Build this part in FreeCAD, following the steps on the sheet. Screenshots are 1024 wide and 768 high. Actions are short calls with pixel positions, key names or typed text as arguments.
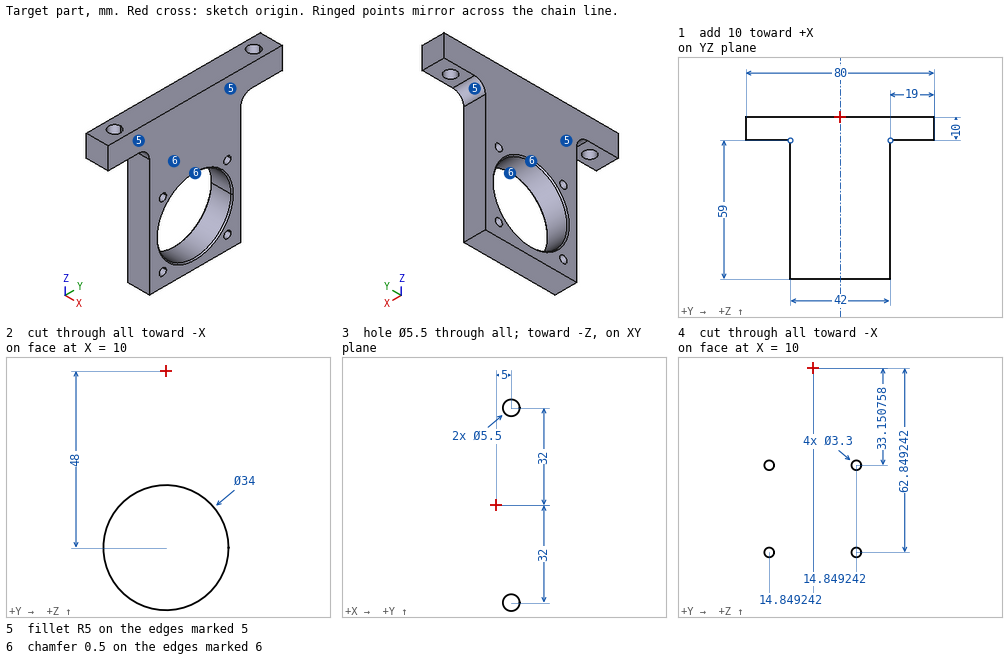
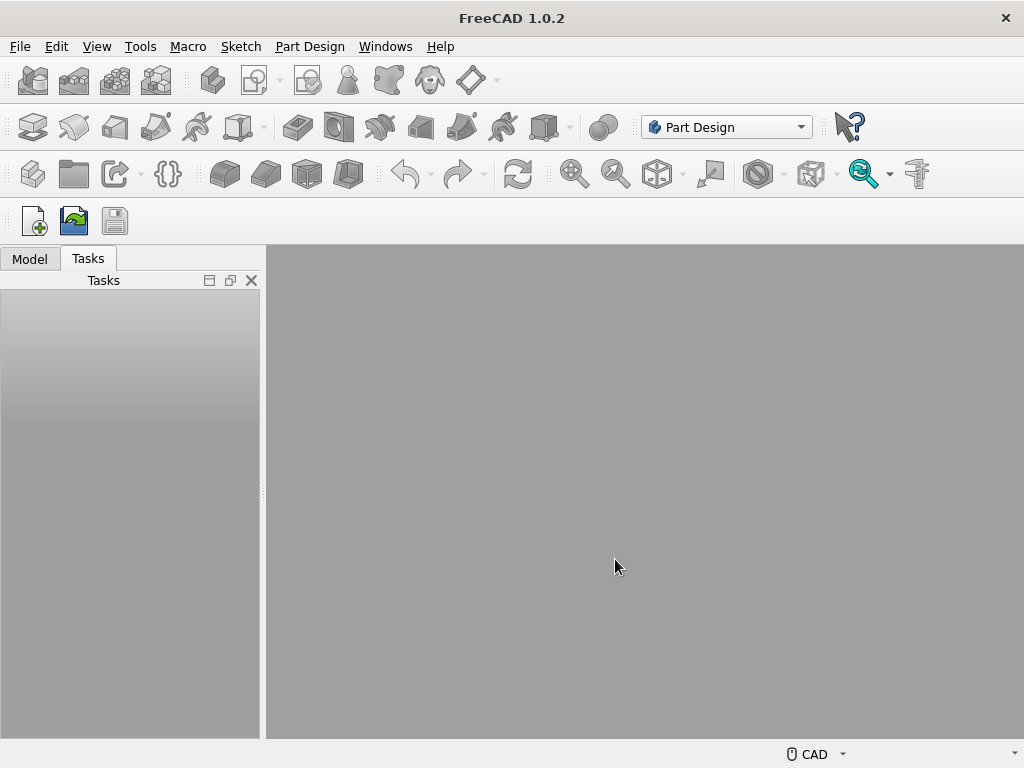
click(33, 222)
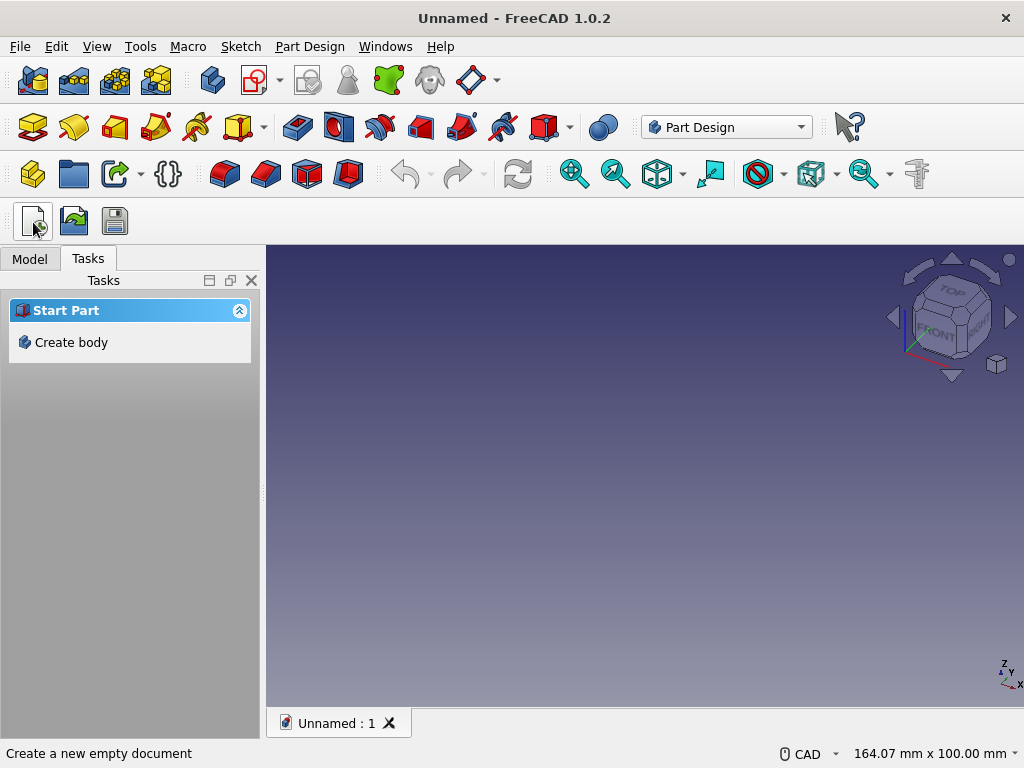
click(254, 80)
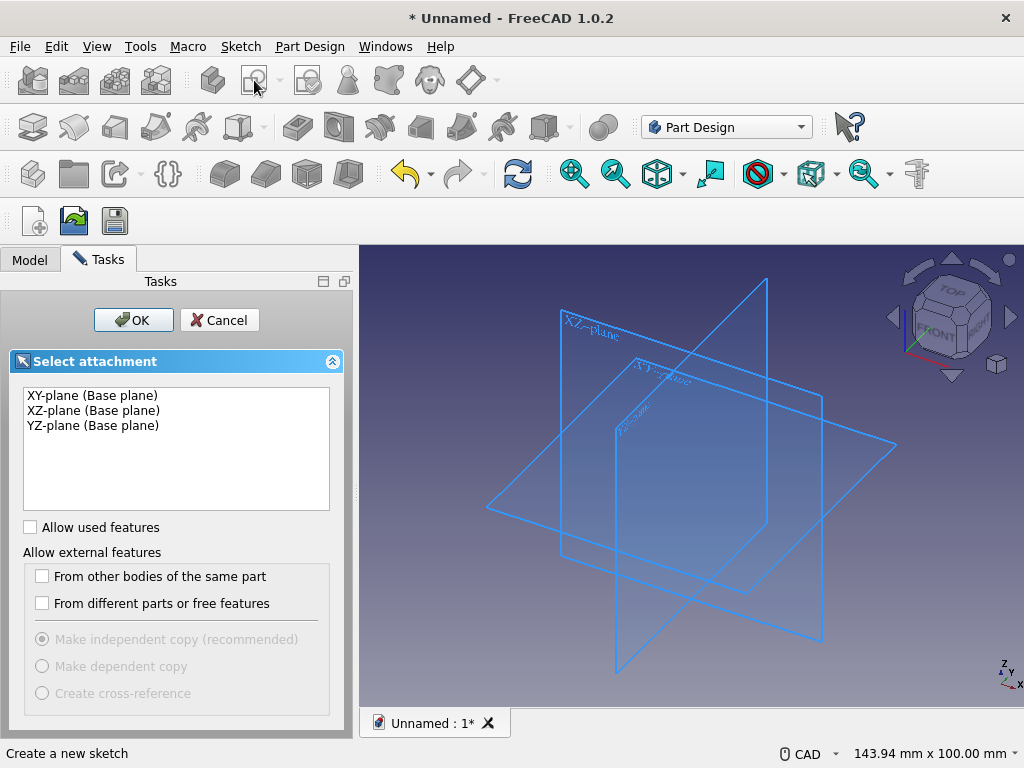
click(84, 426)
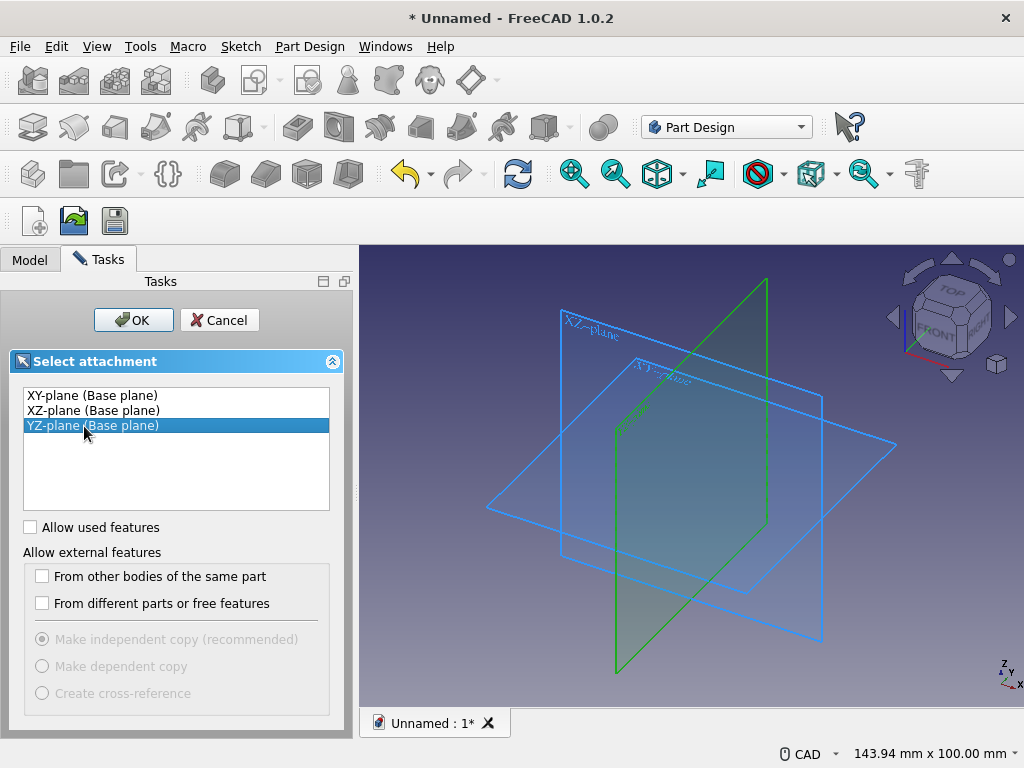
click(134, 320)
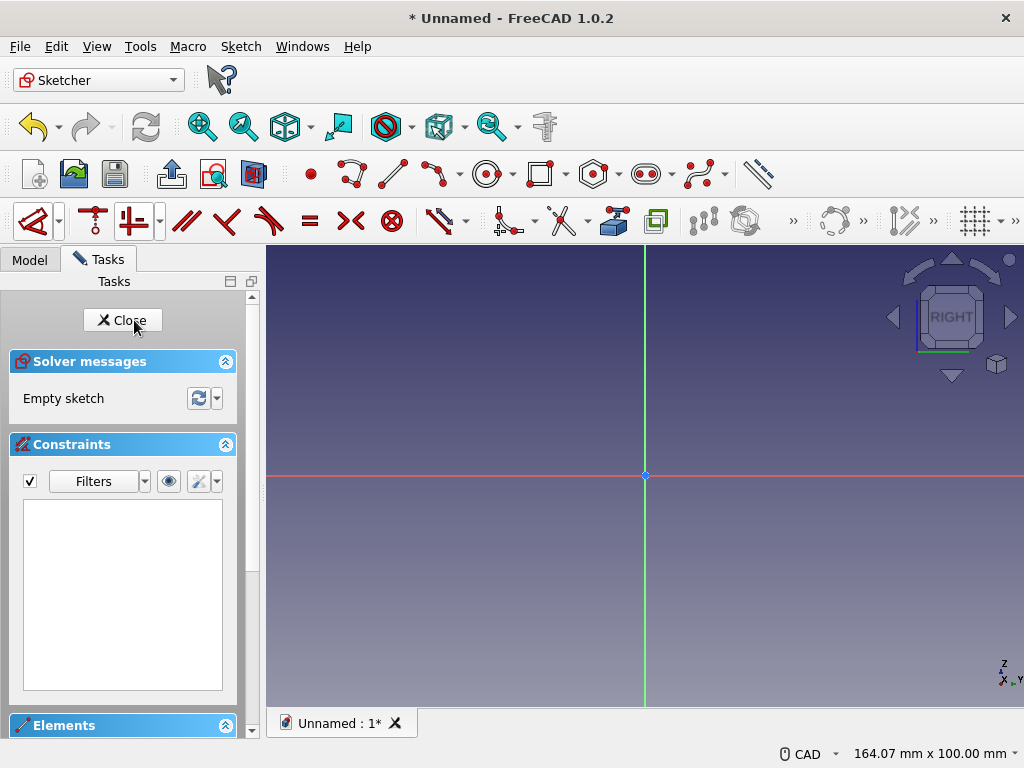
scroll(437, 273, down, 2)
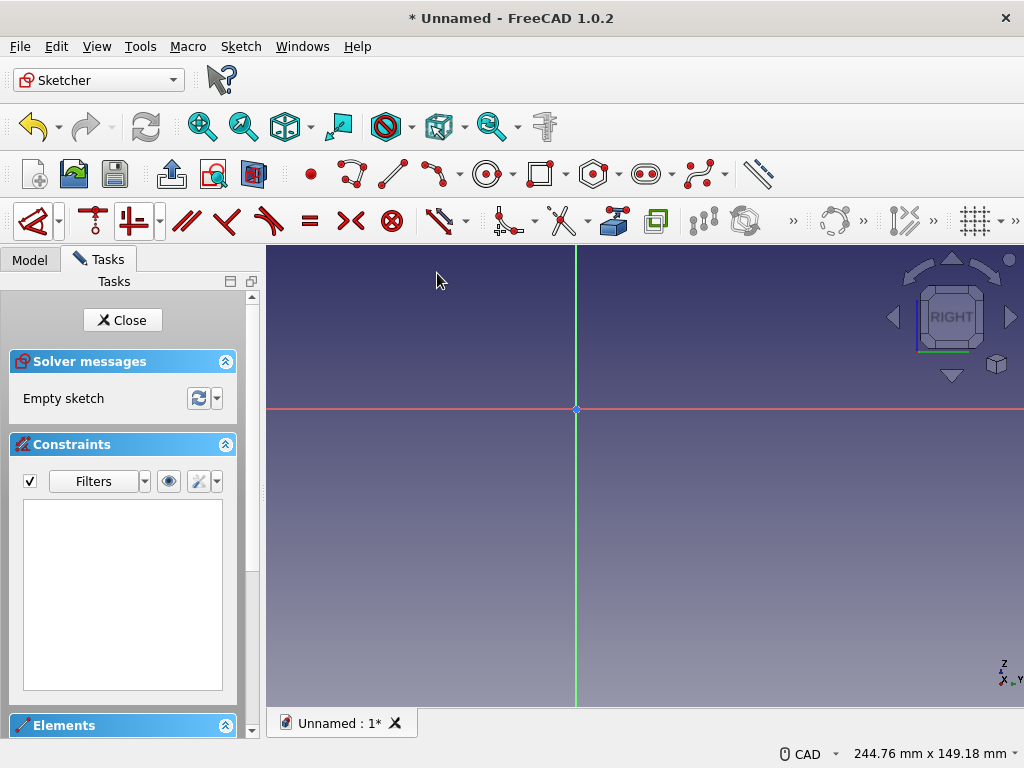
click(352, 174)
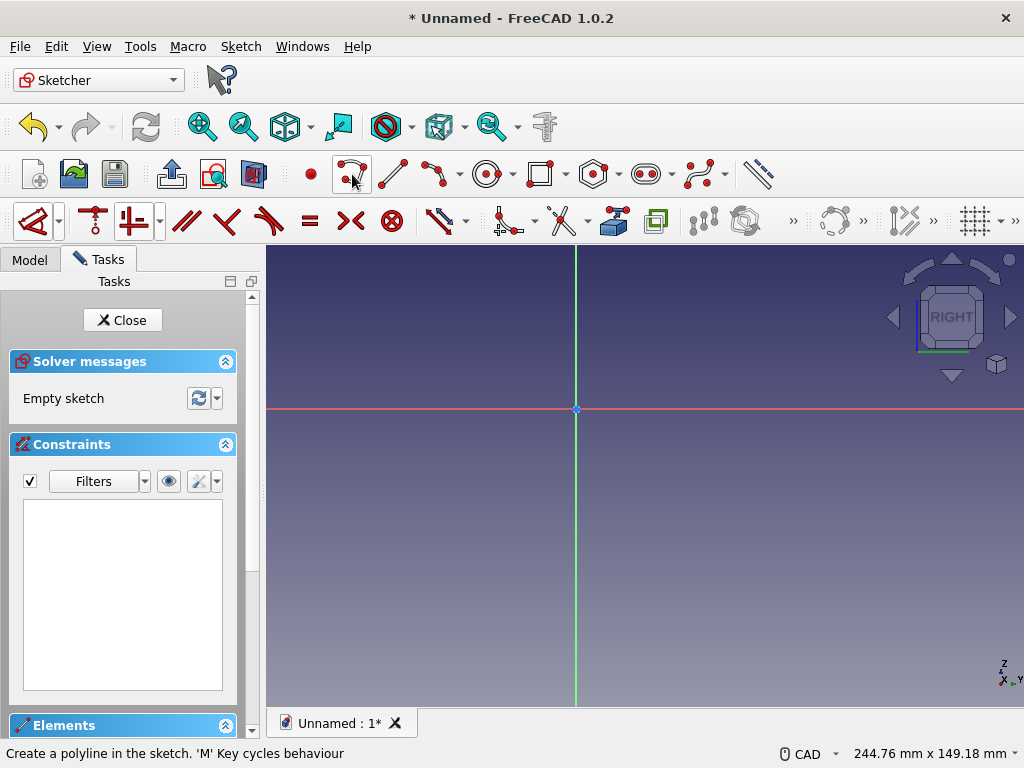
click(511, 440)
click(511, 623)
click(642, 623)
click(642, 440)
click(700, 440)
click(700, 409)
click(453, 418)
click(453, 440)
click(511, 441)
key(Escape)
key(Escape)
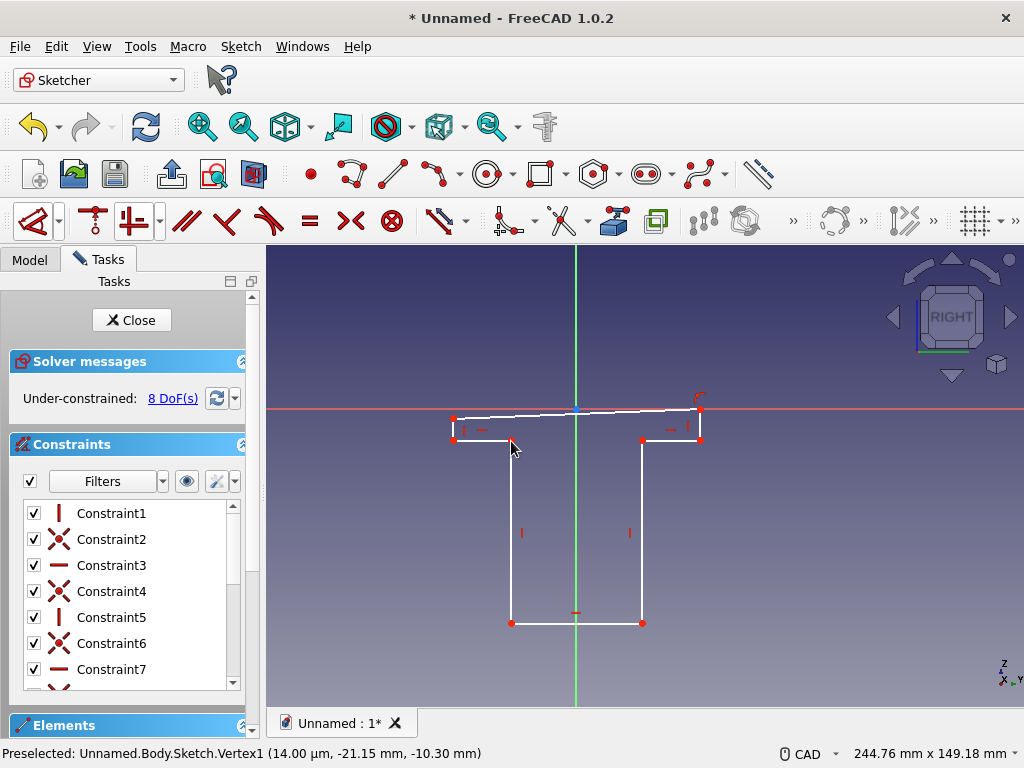
click(626, 412)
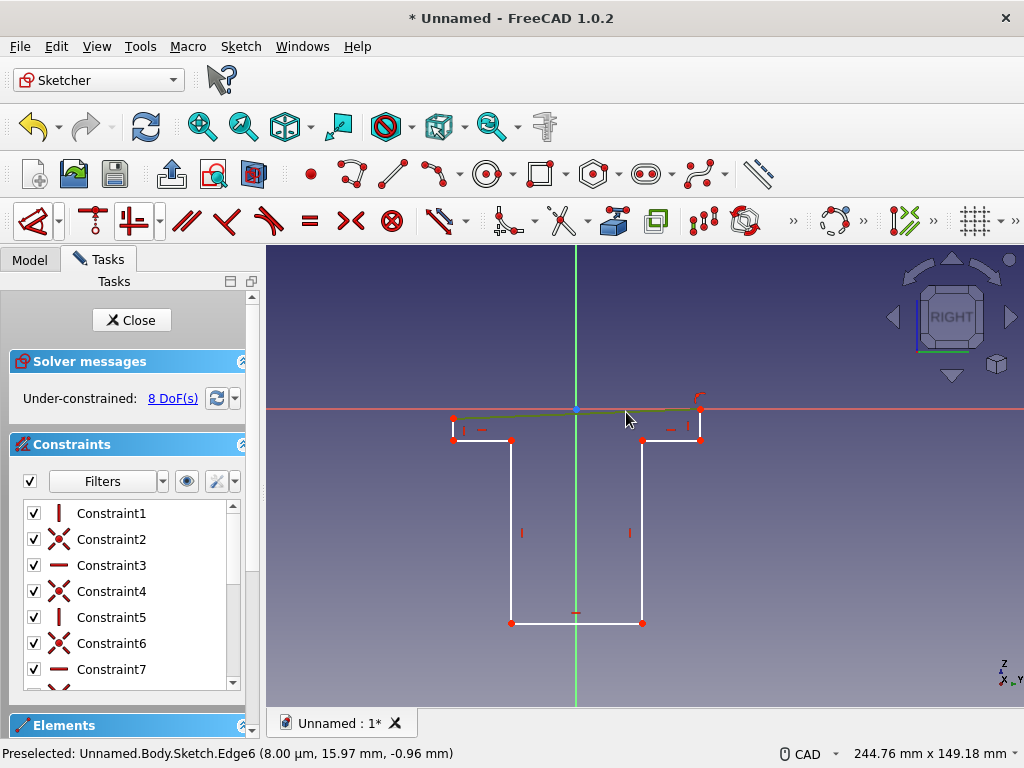
key(h)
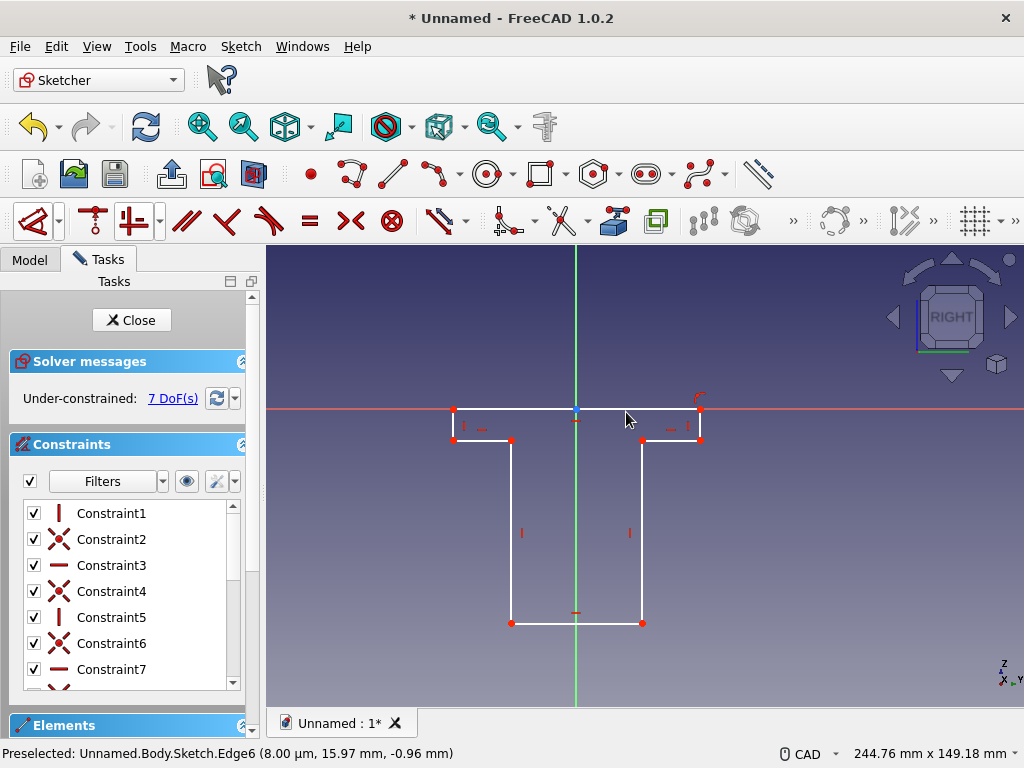
click(511, 441)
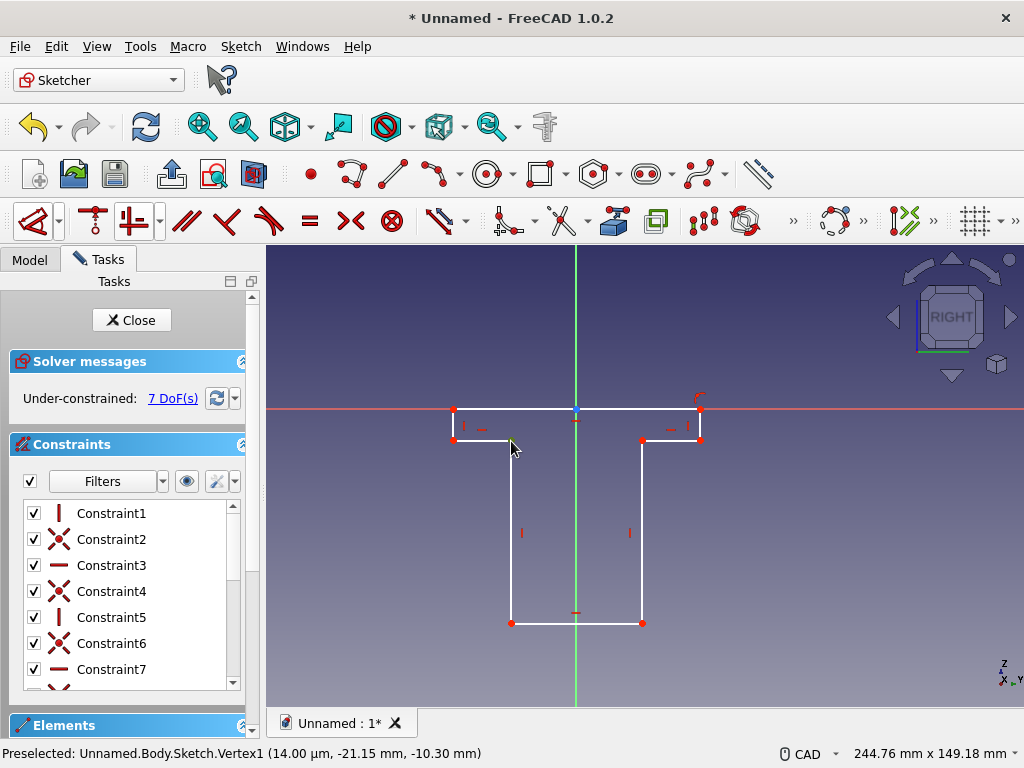
click(642, 441)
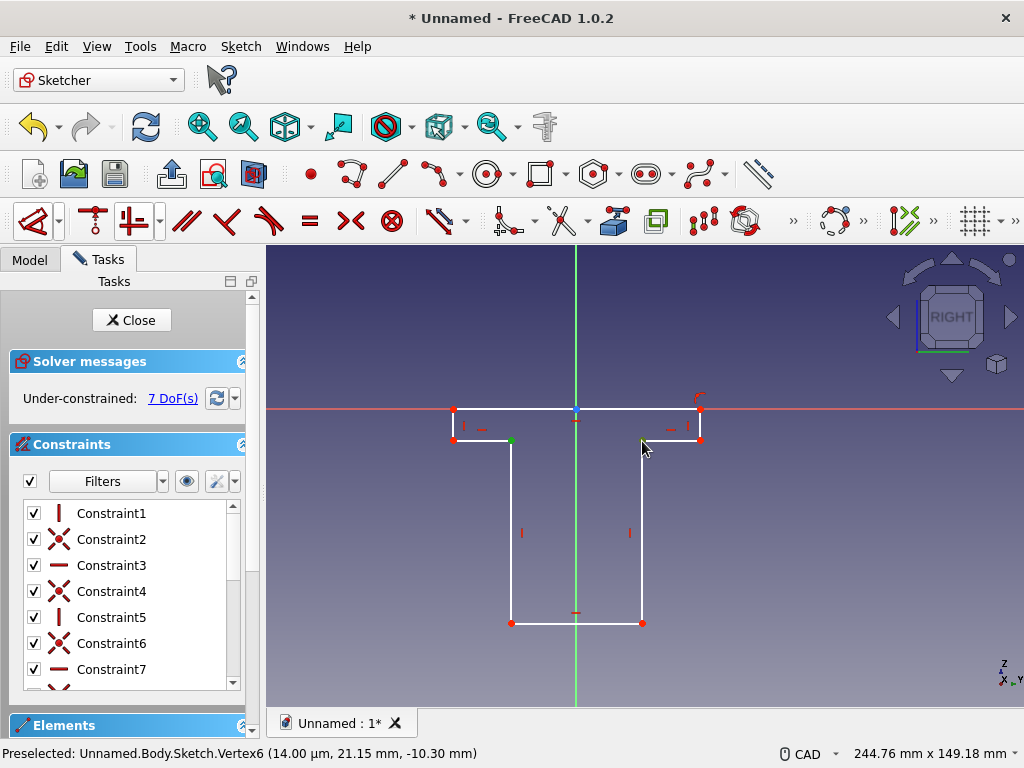
click(577, 592)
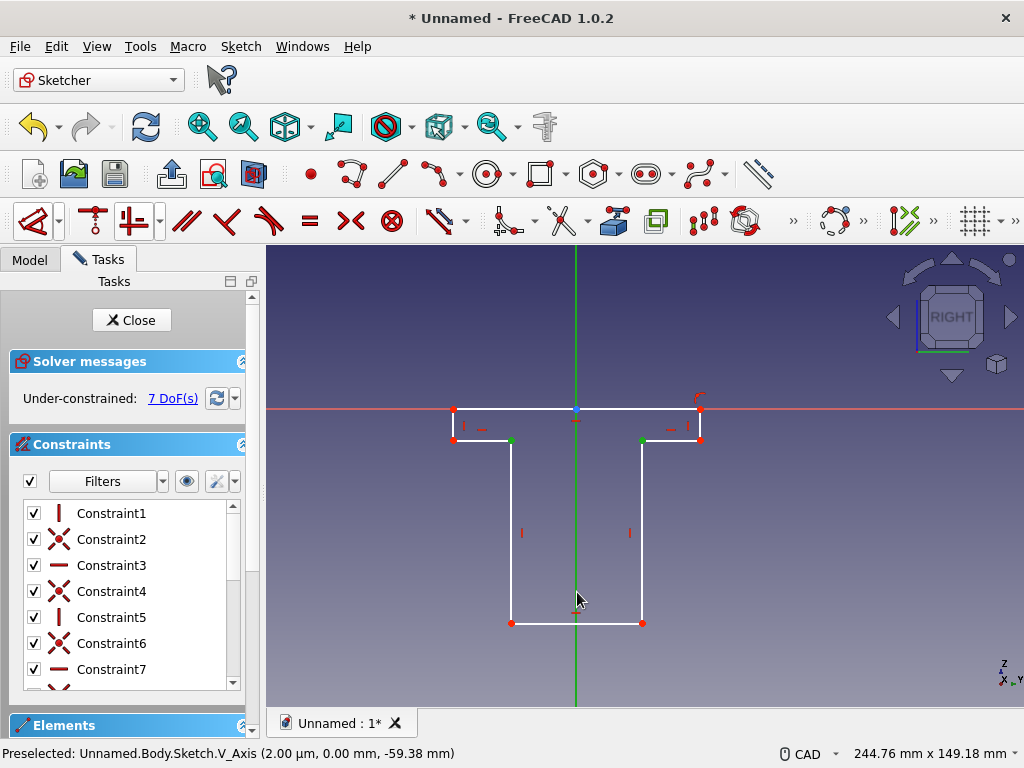
click(351, 222)